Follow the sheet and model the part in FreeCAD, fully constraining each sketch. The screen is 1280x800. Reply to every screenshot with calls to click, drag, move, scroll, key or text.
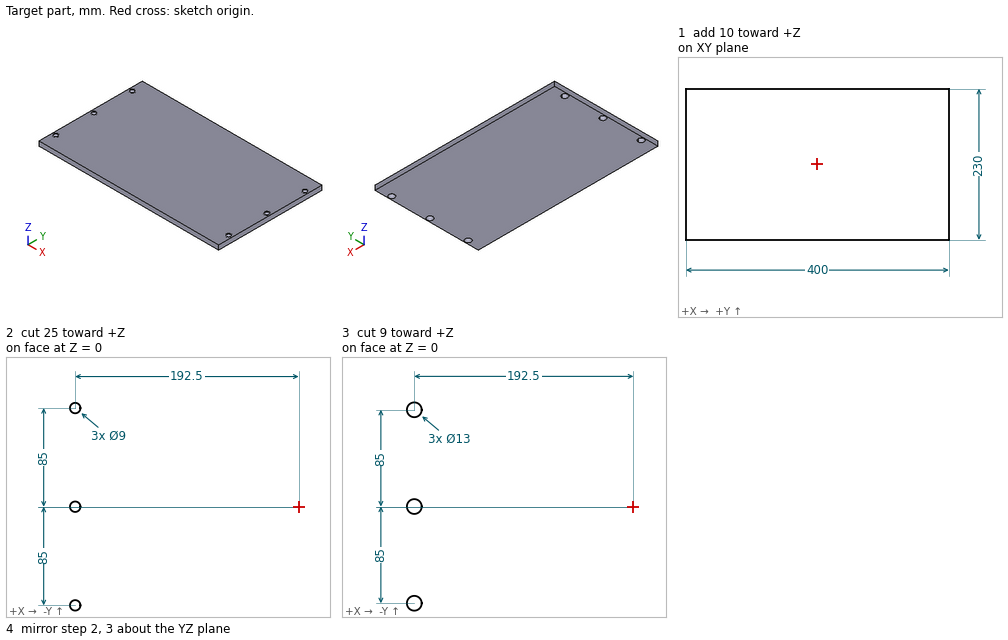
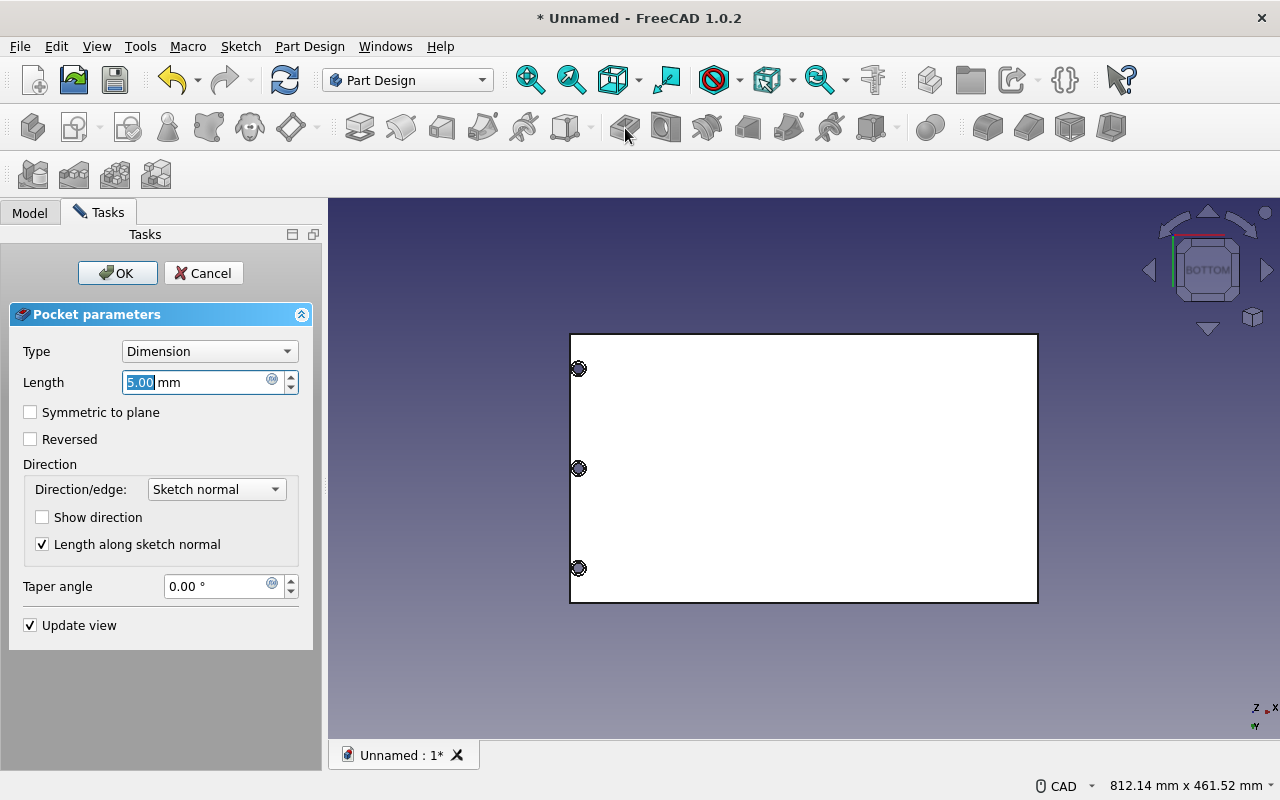
text(9)
key(Tab)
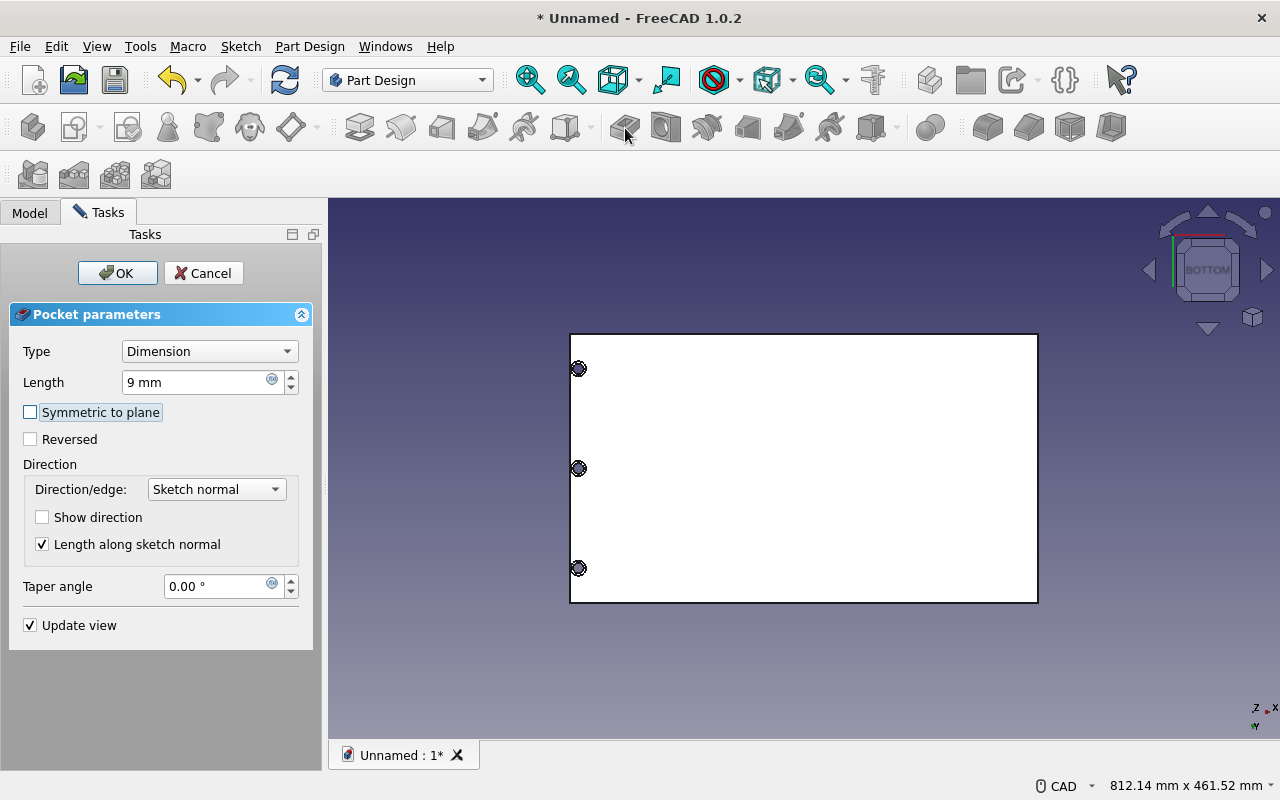
click(118, 273)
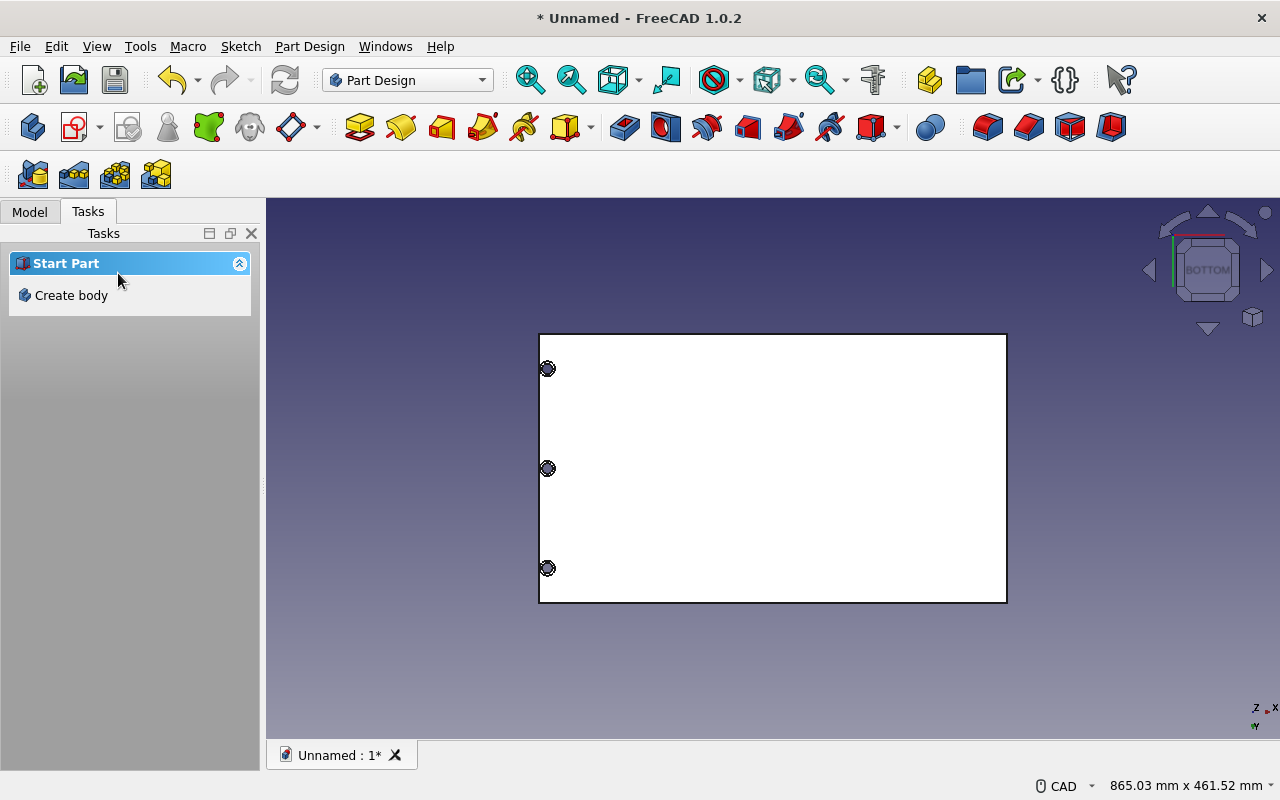
click(30, 212)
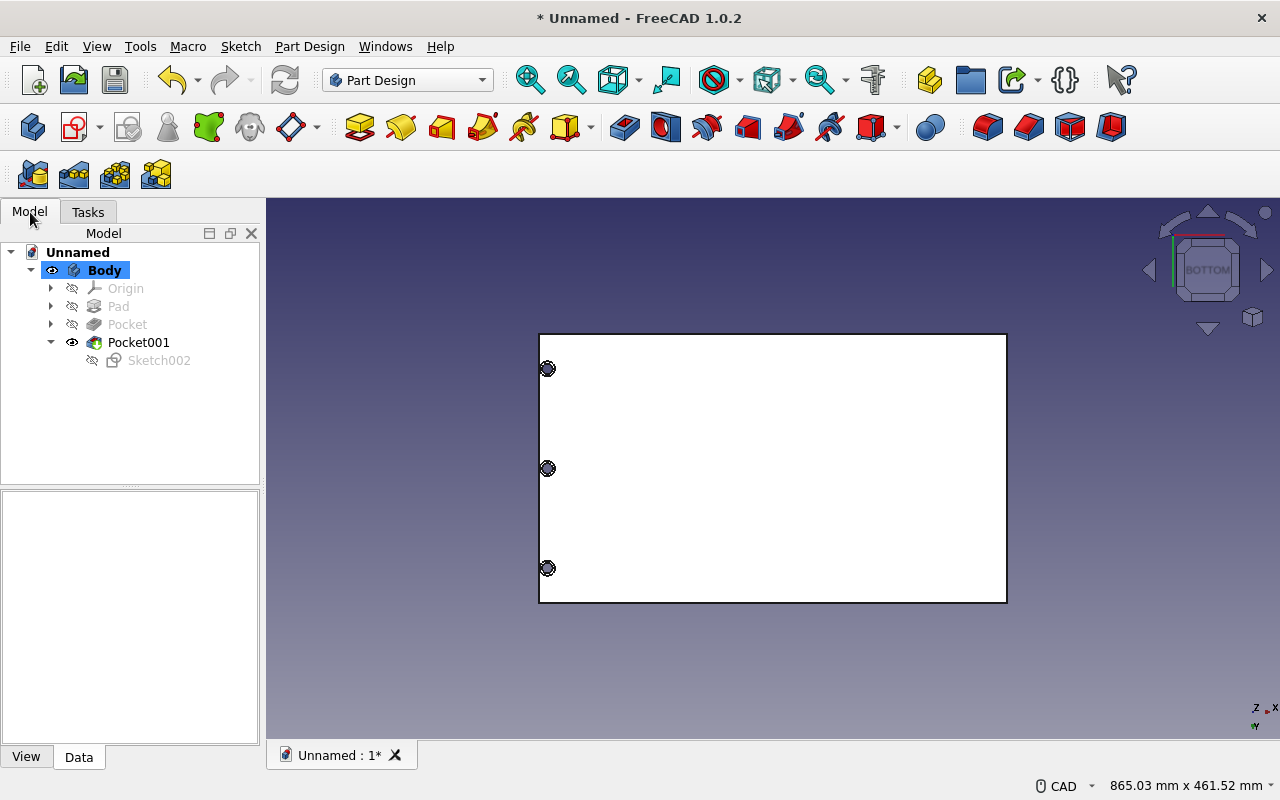
click(117, 324)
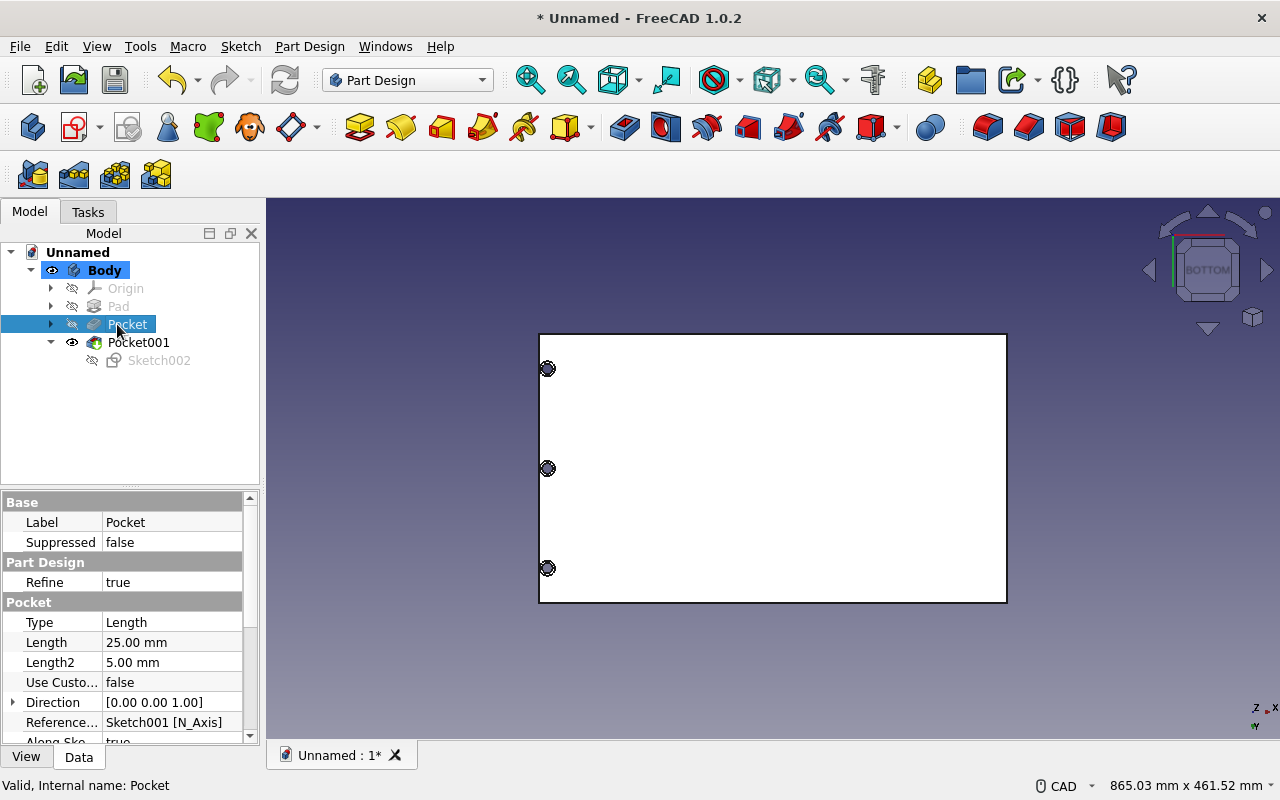
click(117, 342, ctrl)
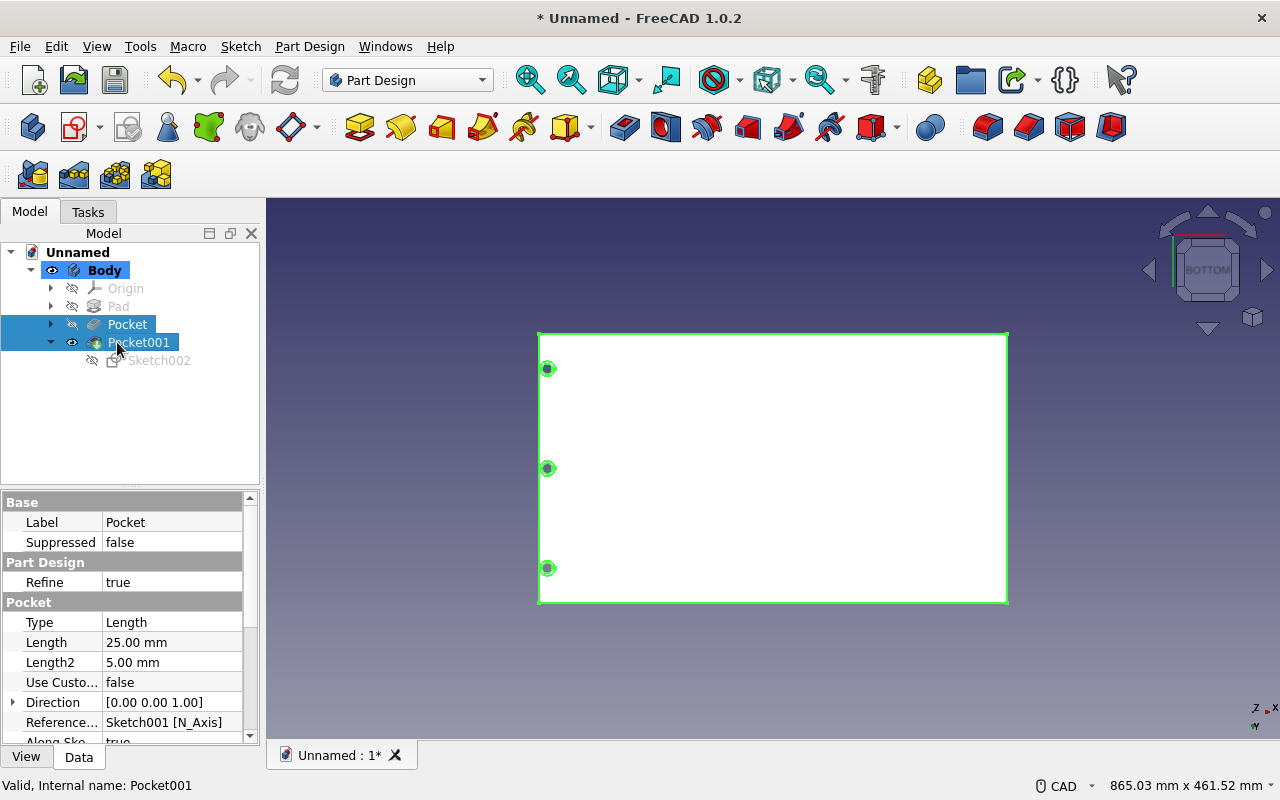
click(33, 174)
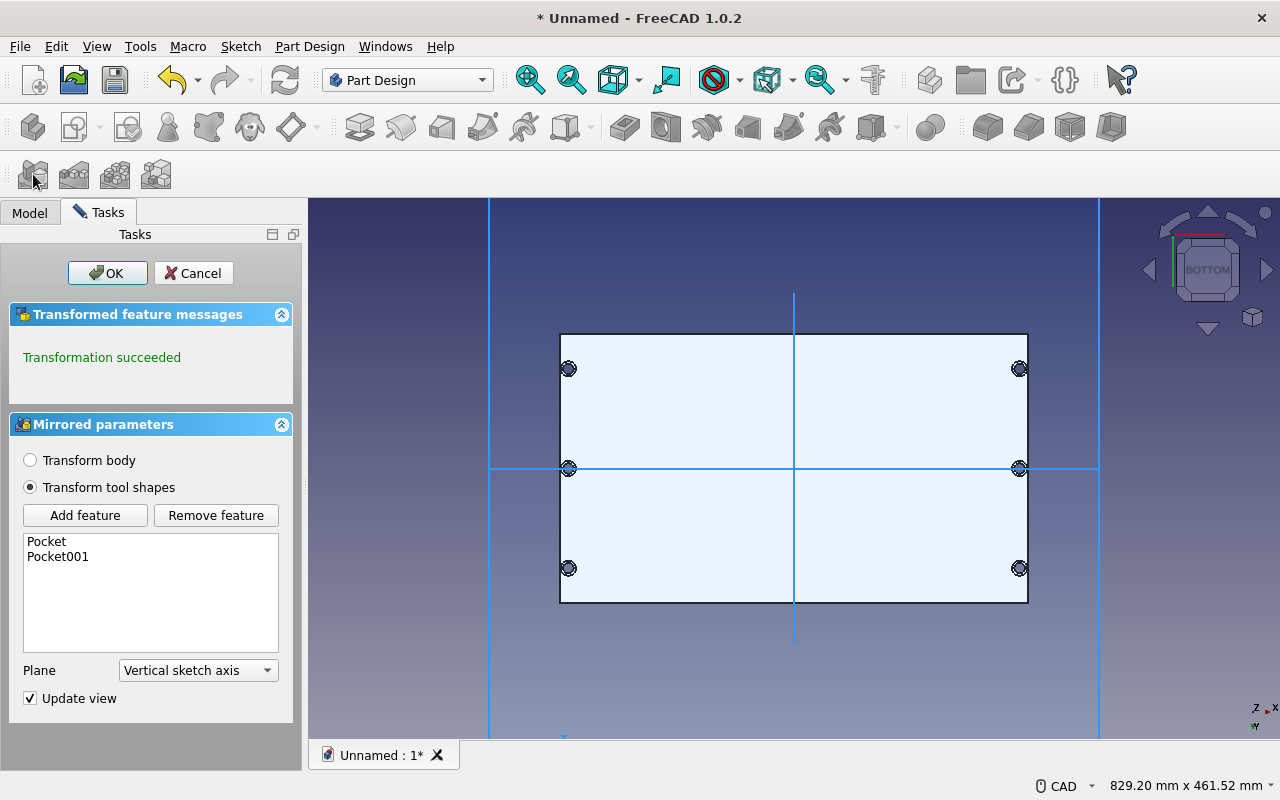
click(199, 670)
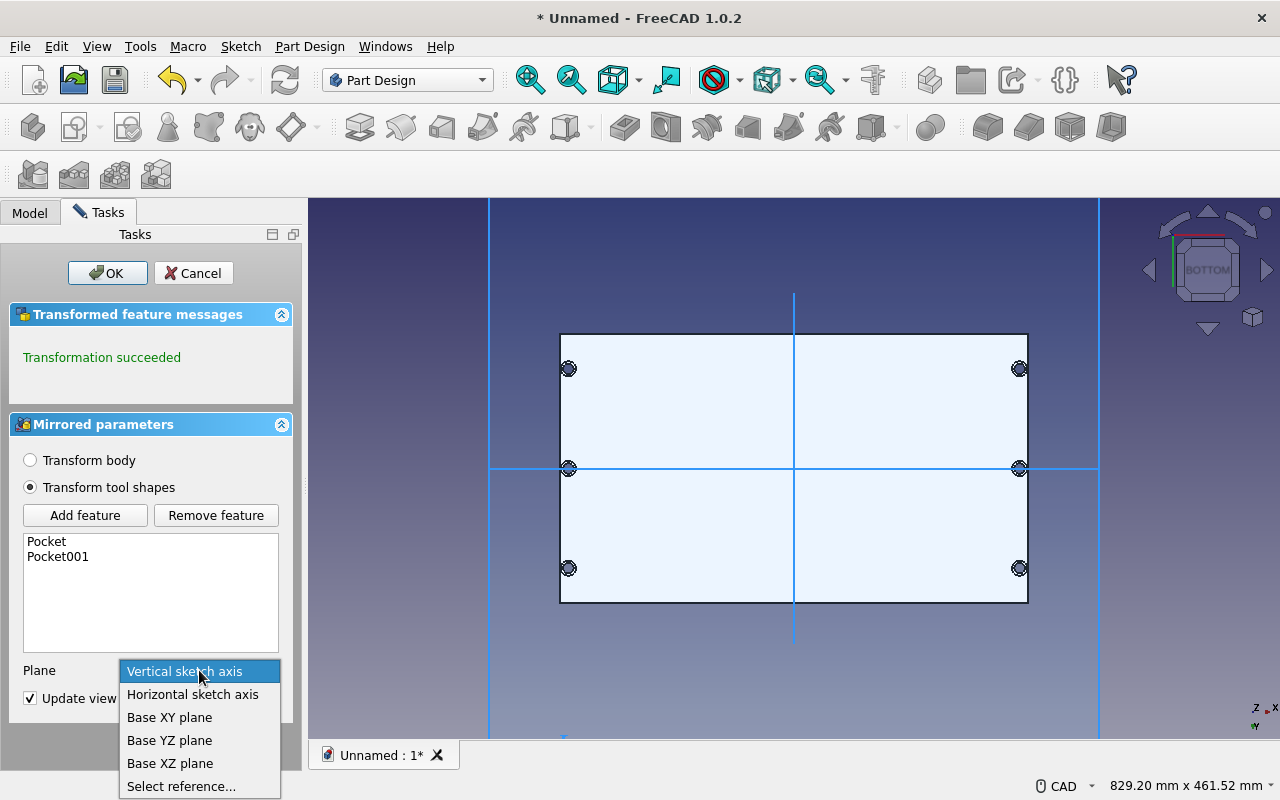
click(198, 740)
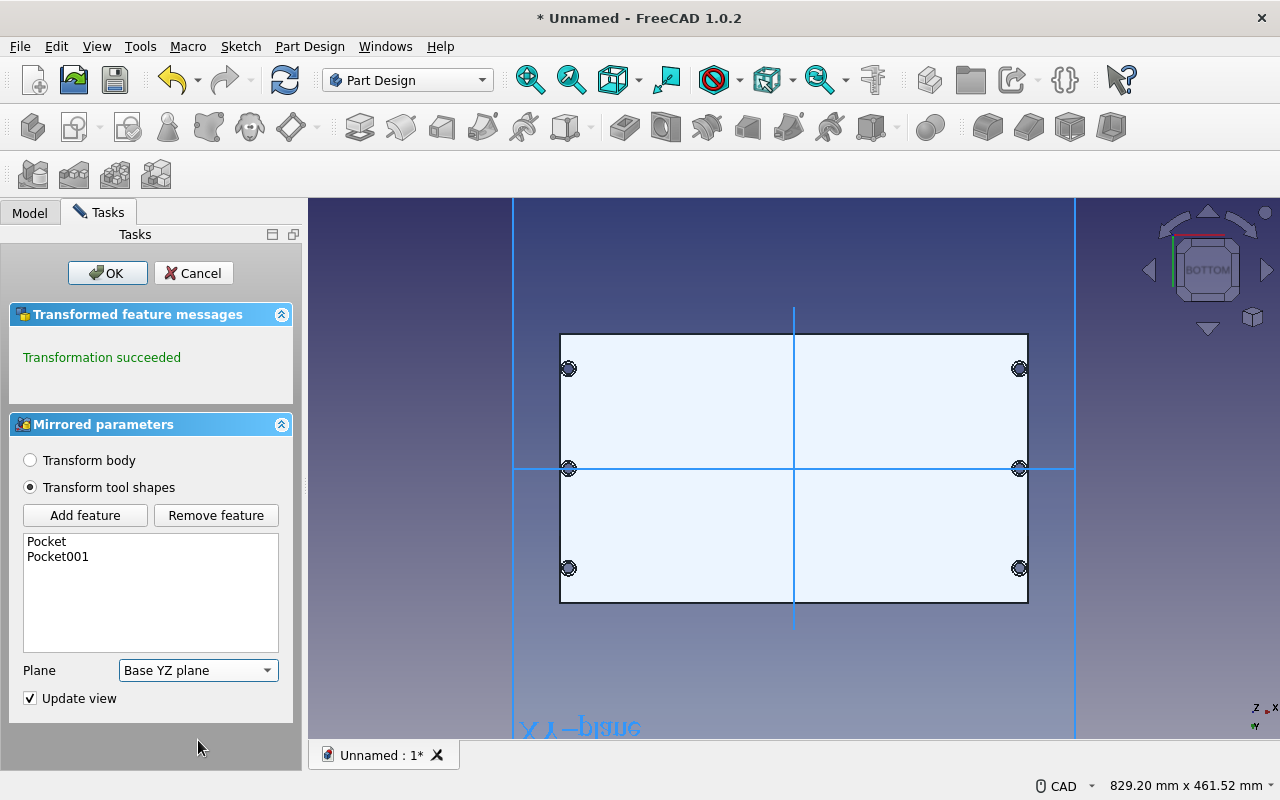
click(108, 273)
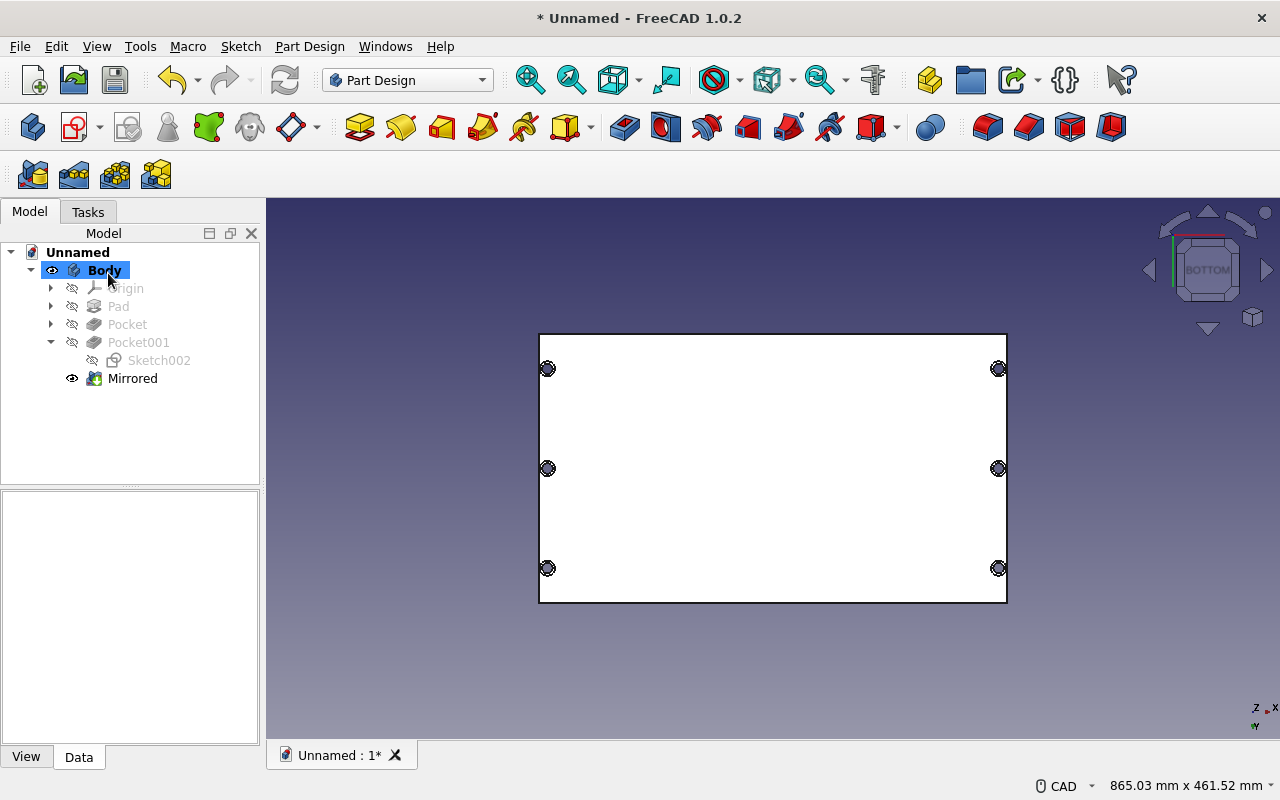
key(0)